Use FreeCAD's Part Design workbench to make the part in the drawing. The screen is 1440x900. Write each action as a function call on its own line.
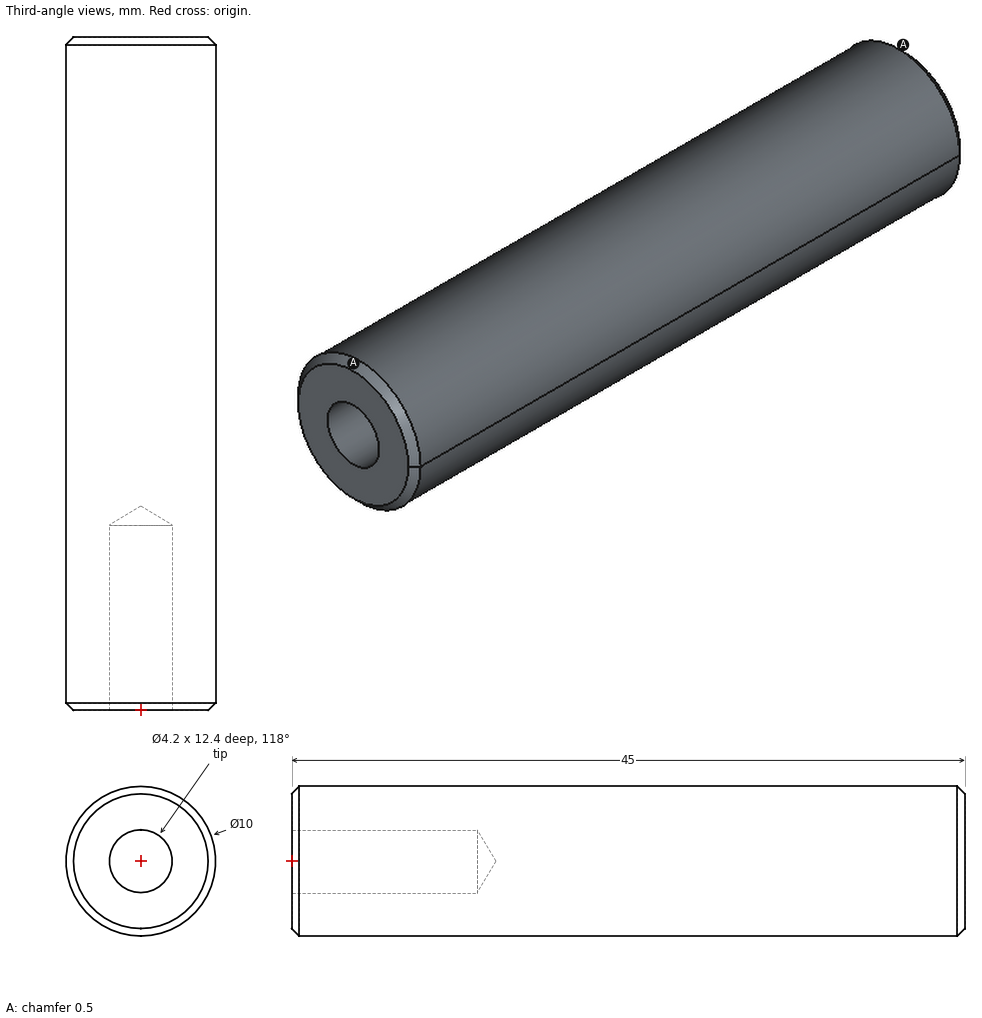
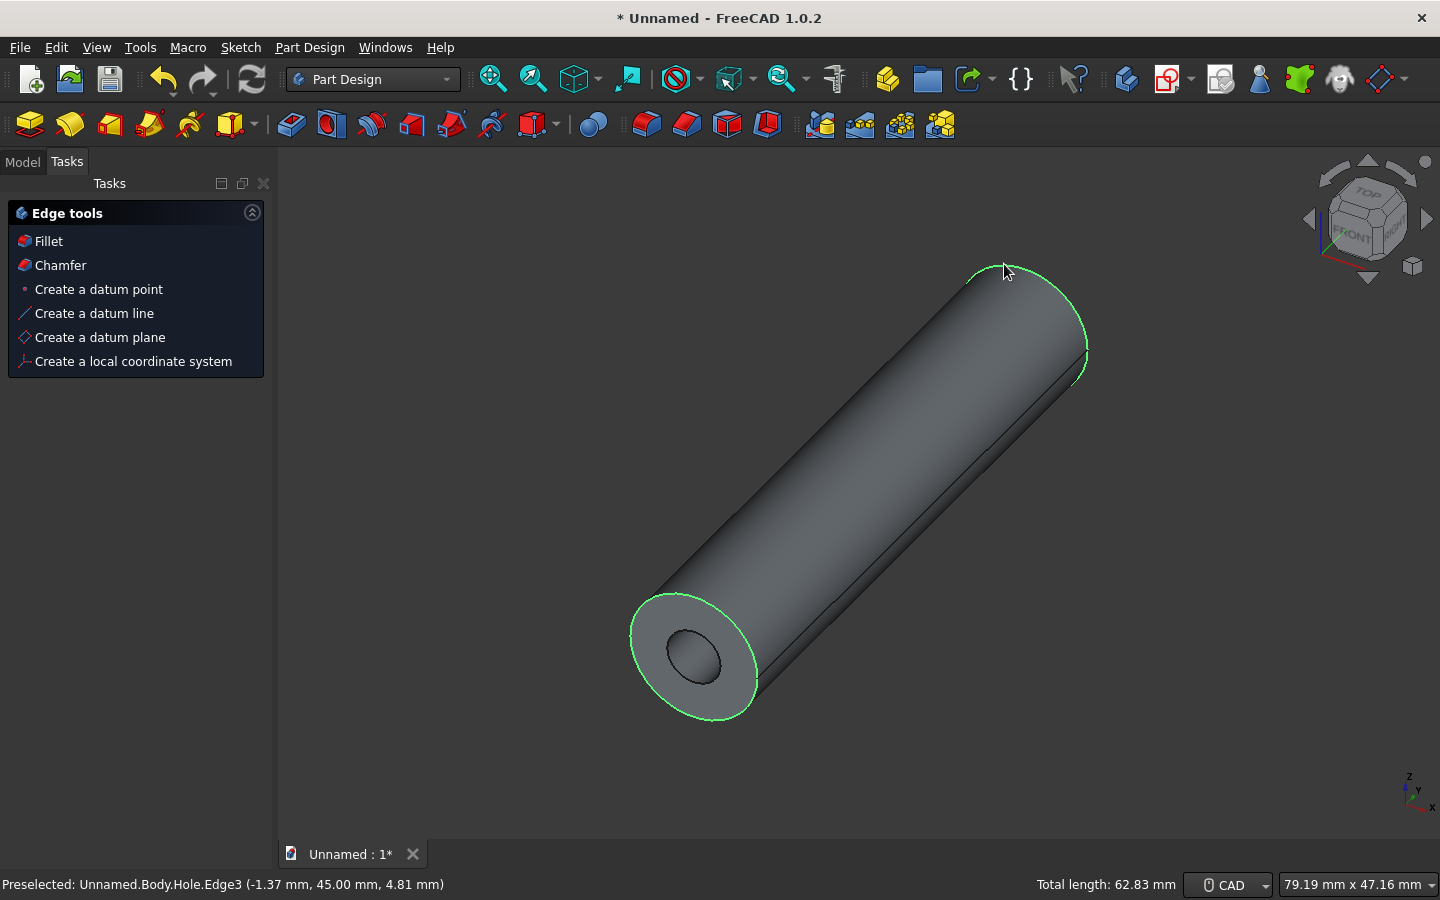
click(688, 124)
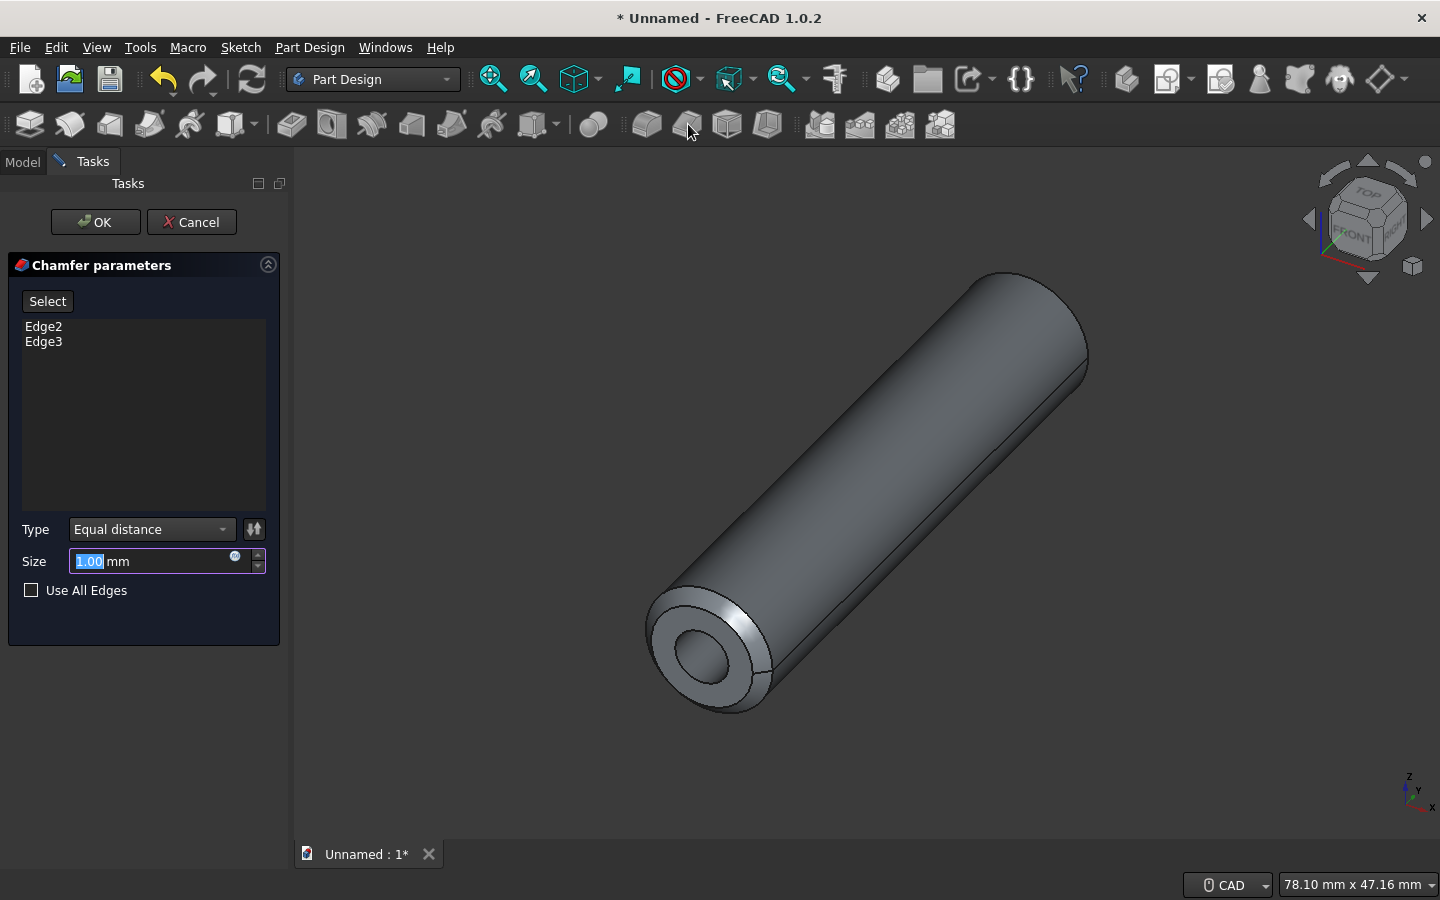
text(0.5)
key(Tab)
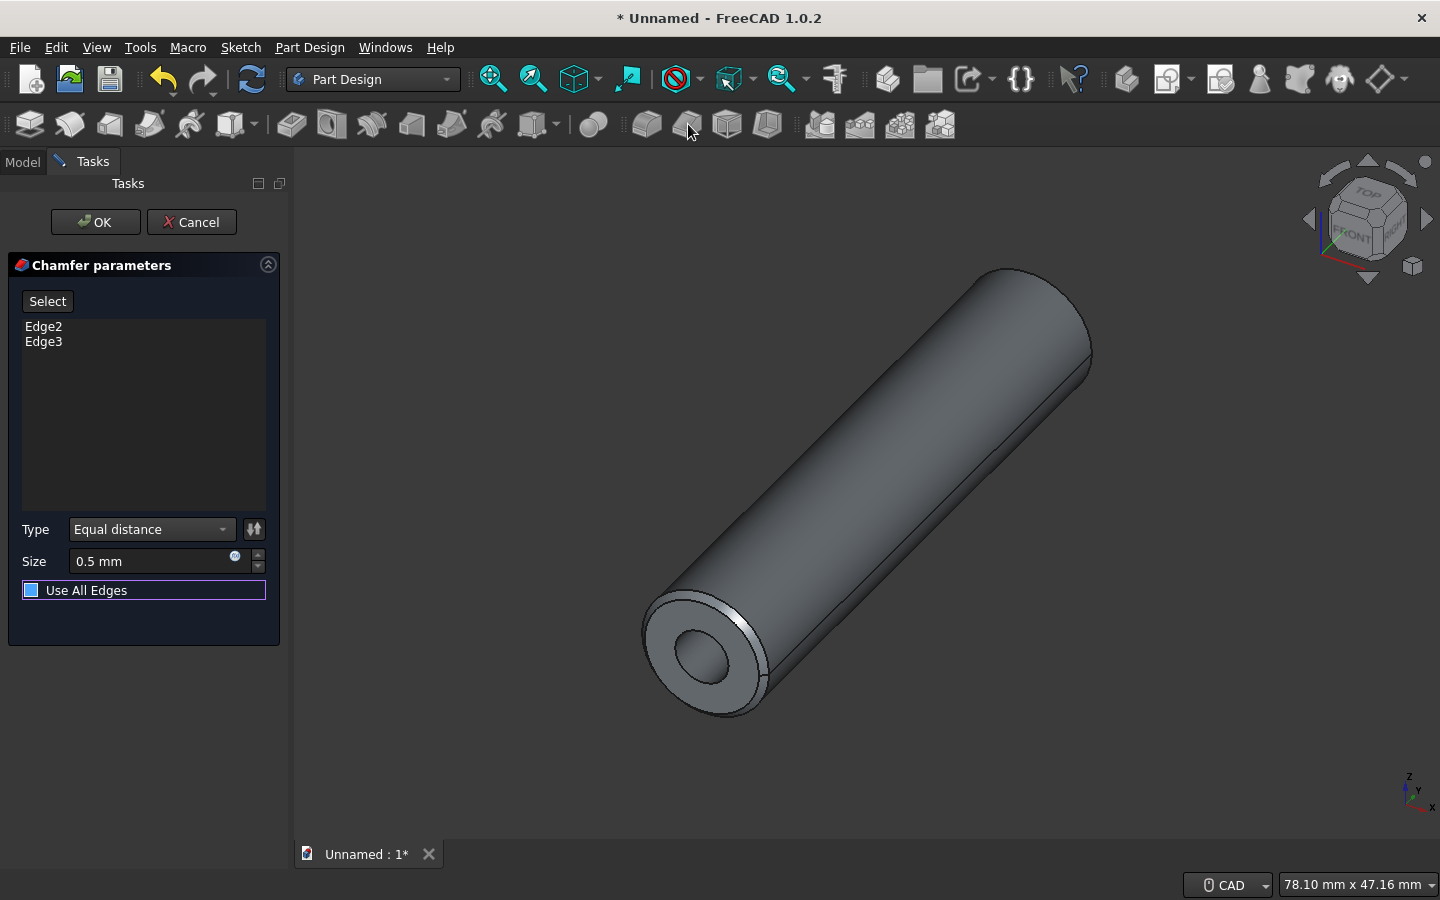
click(96, 222)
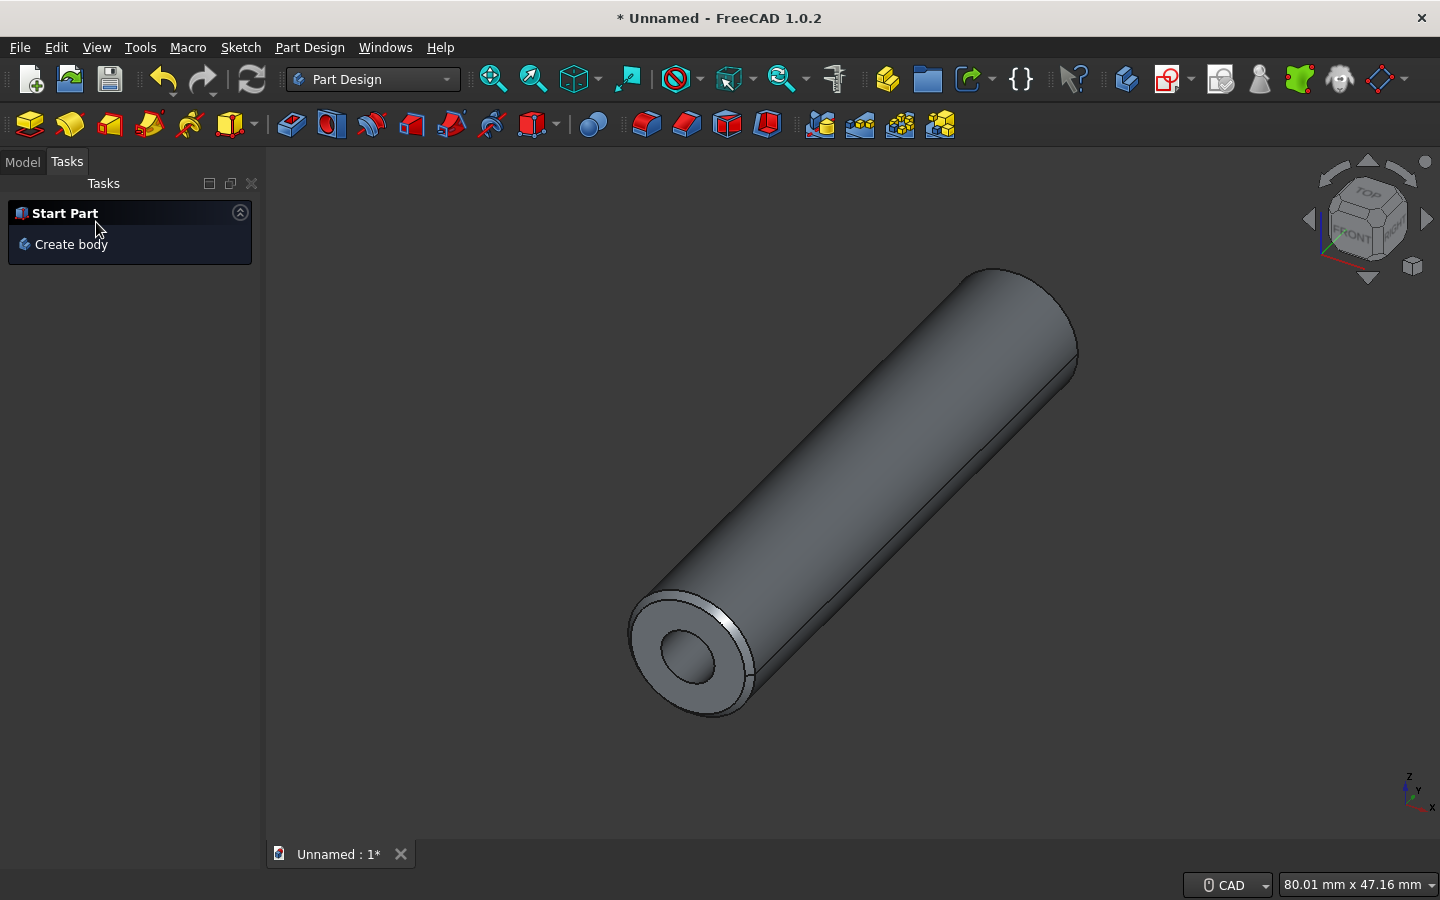
key(0)